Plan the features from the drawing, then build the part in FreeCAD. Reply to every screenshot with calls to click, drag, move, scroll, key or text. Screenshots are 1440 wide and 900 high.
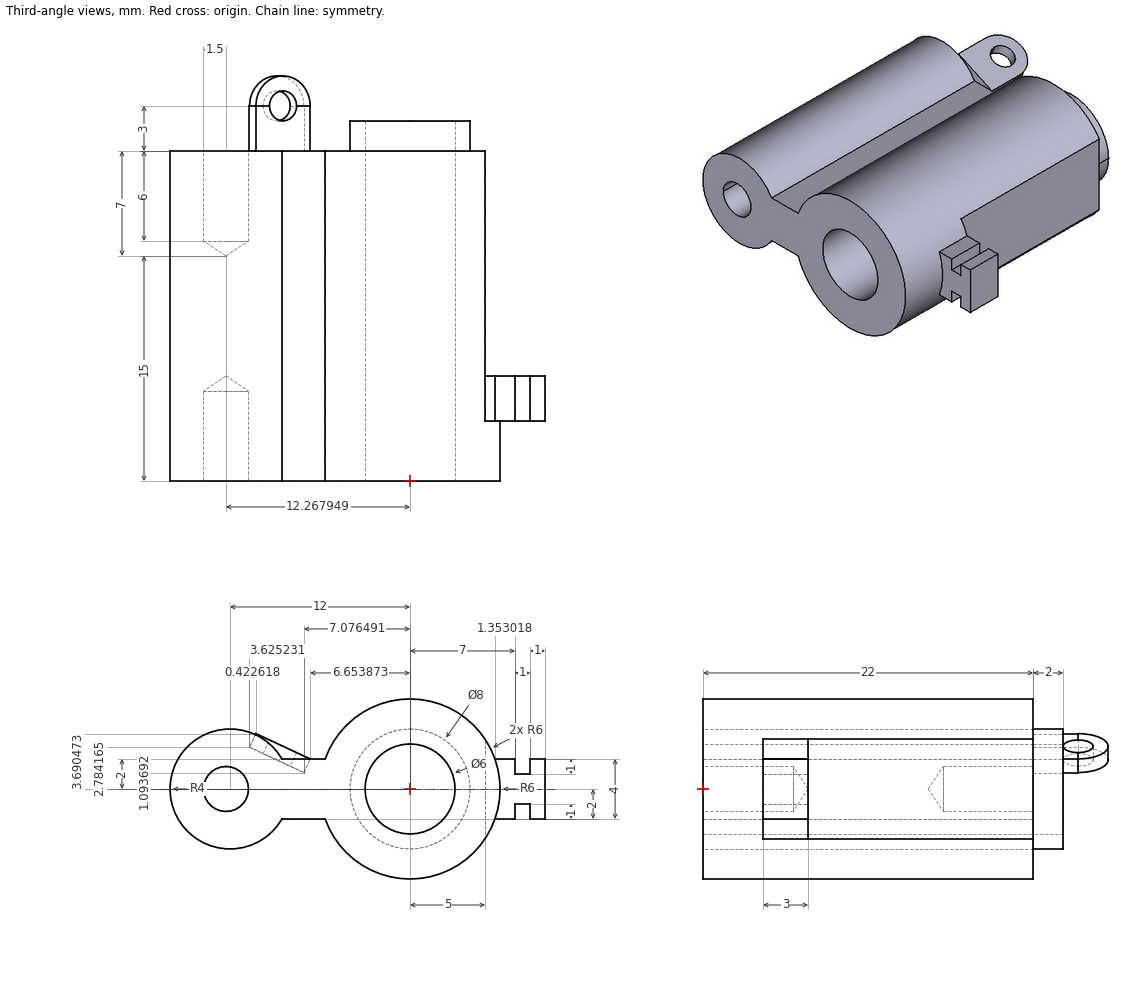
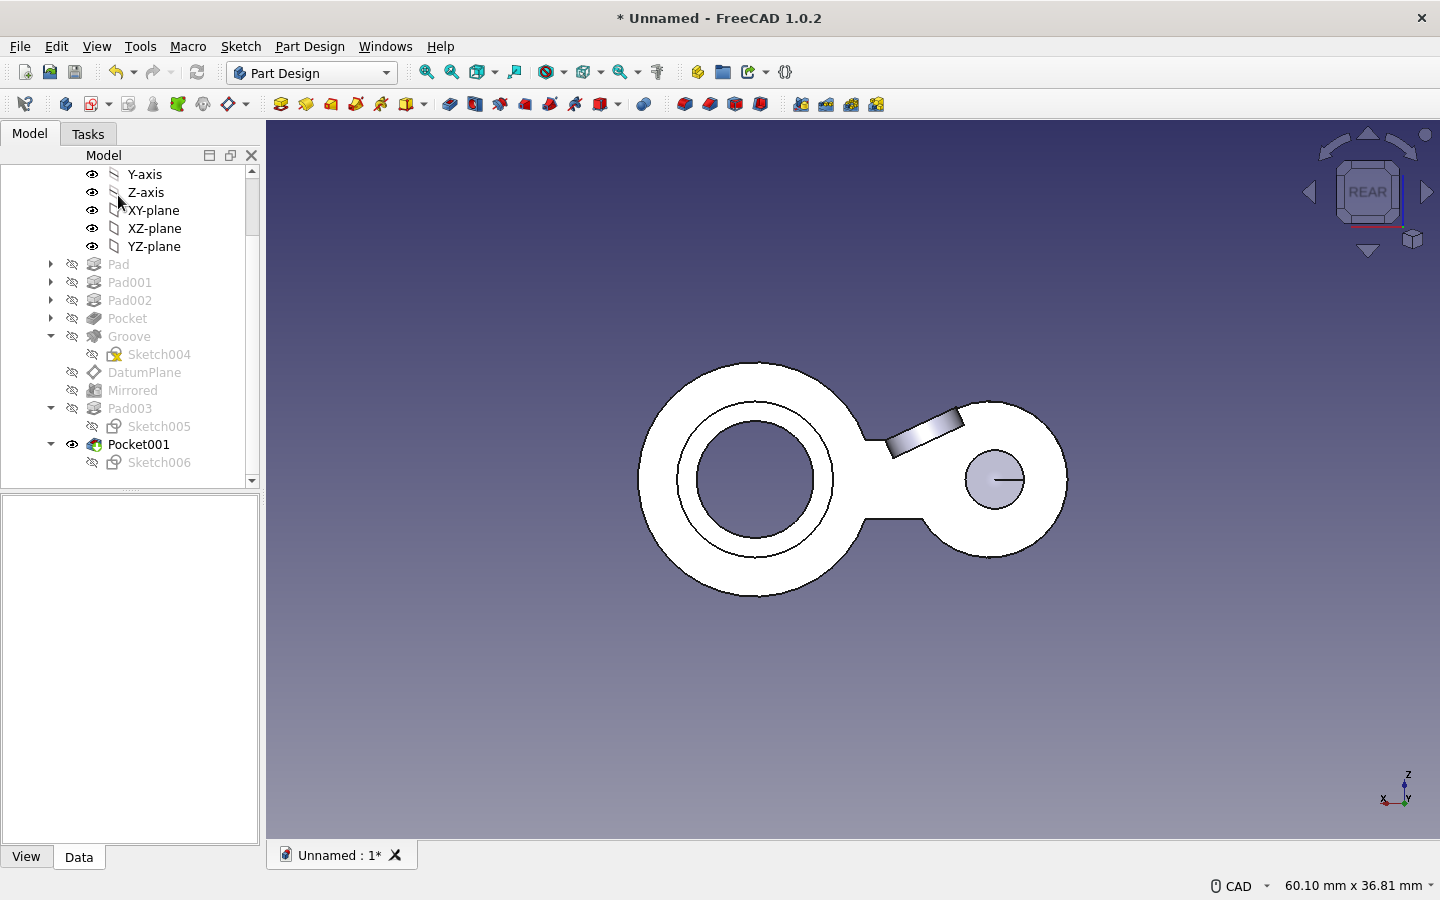
click(427, 72)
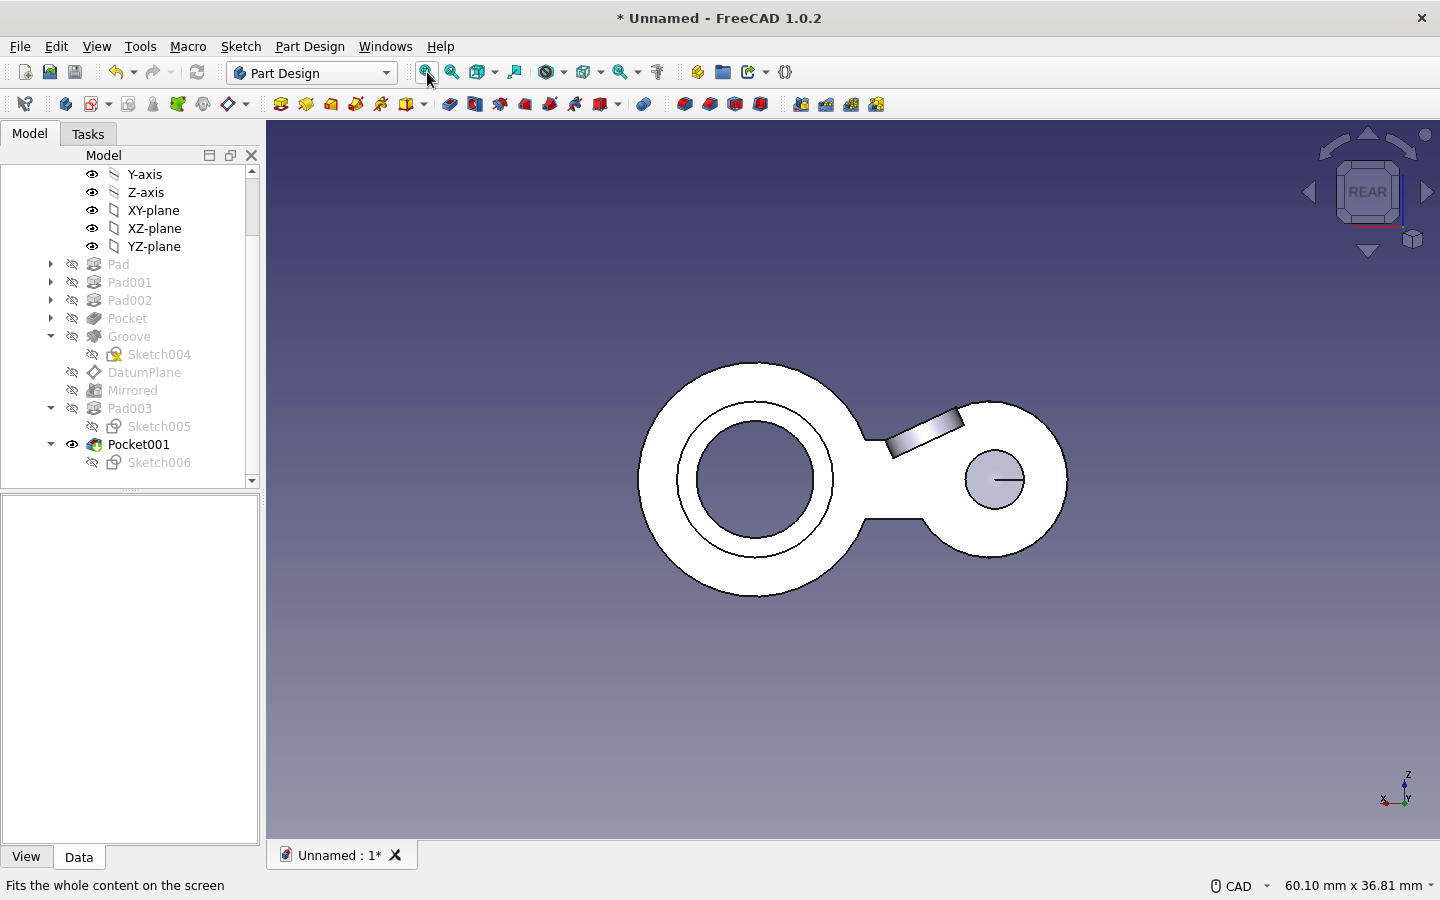
scroll(161, 314, down, 3)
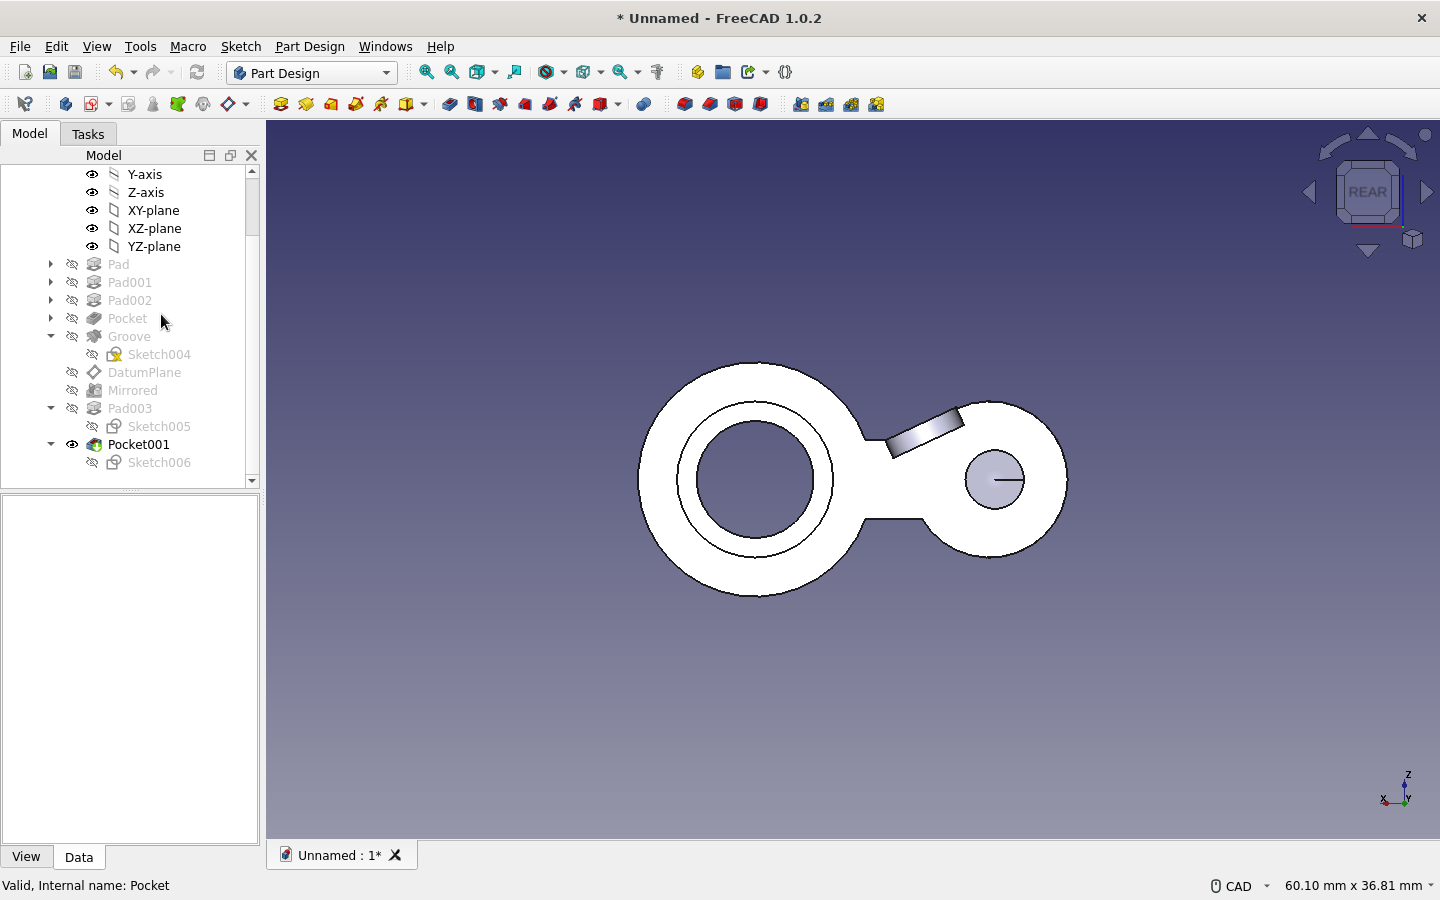
scroll(161, 314, up, 15)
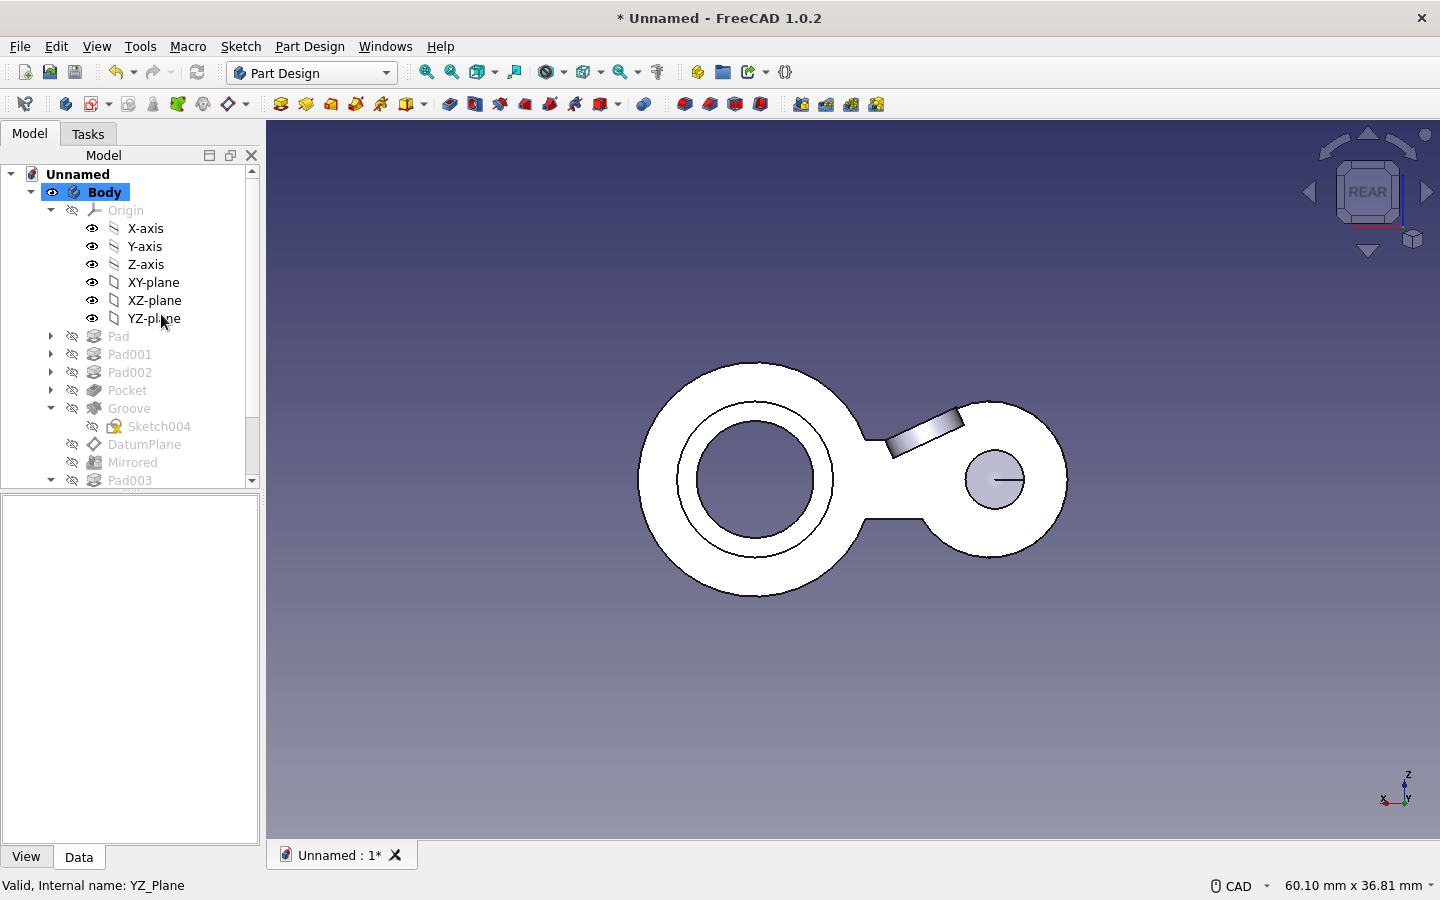
click(137, 300)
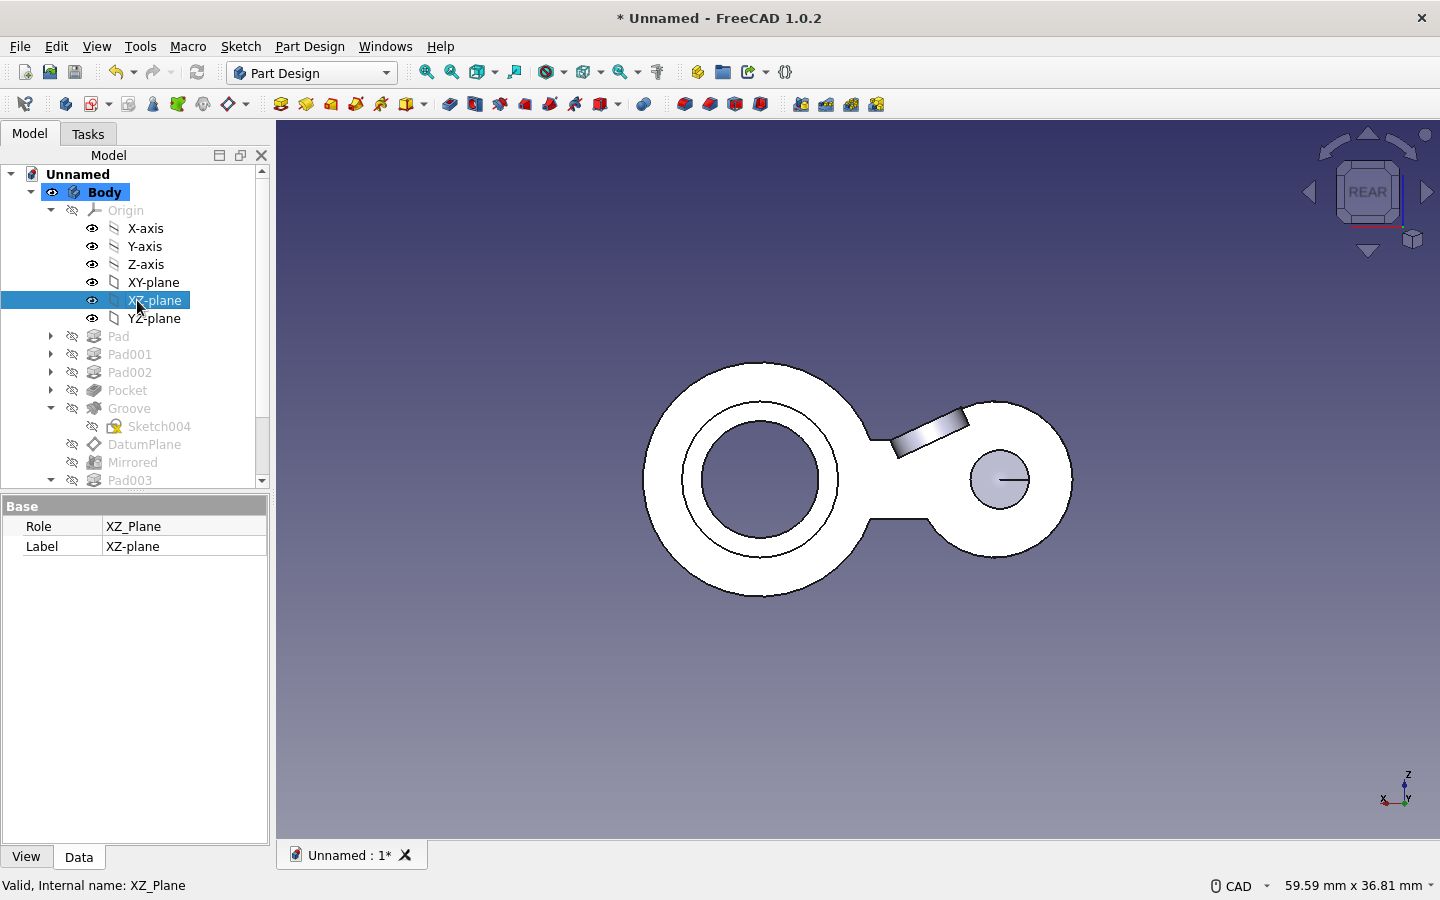
click(228, 104)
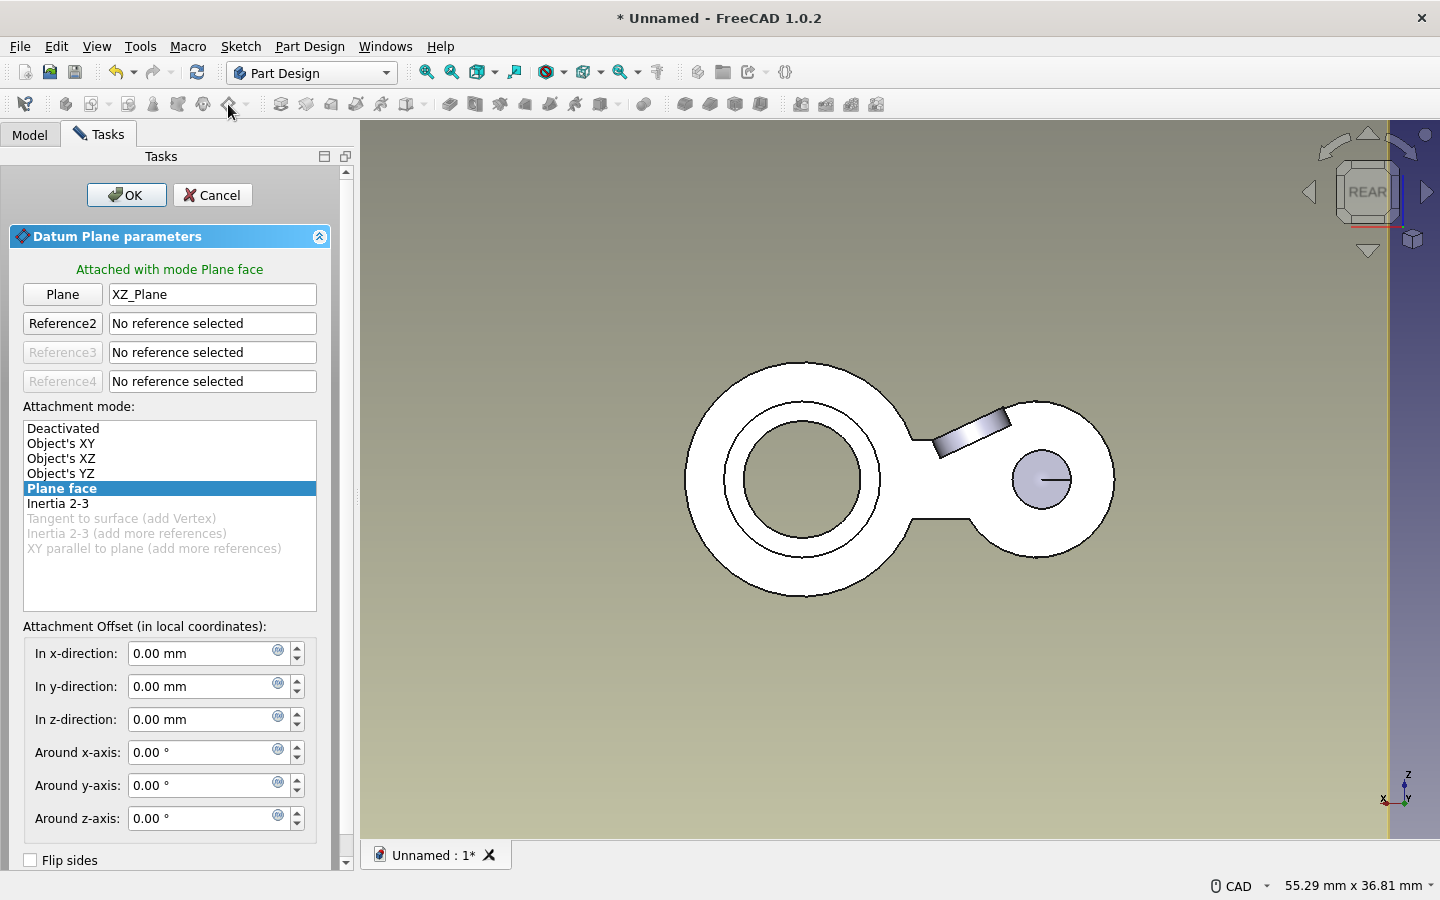
triple_click(210, 720)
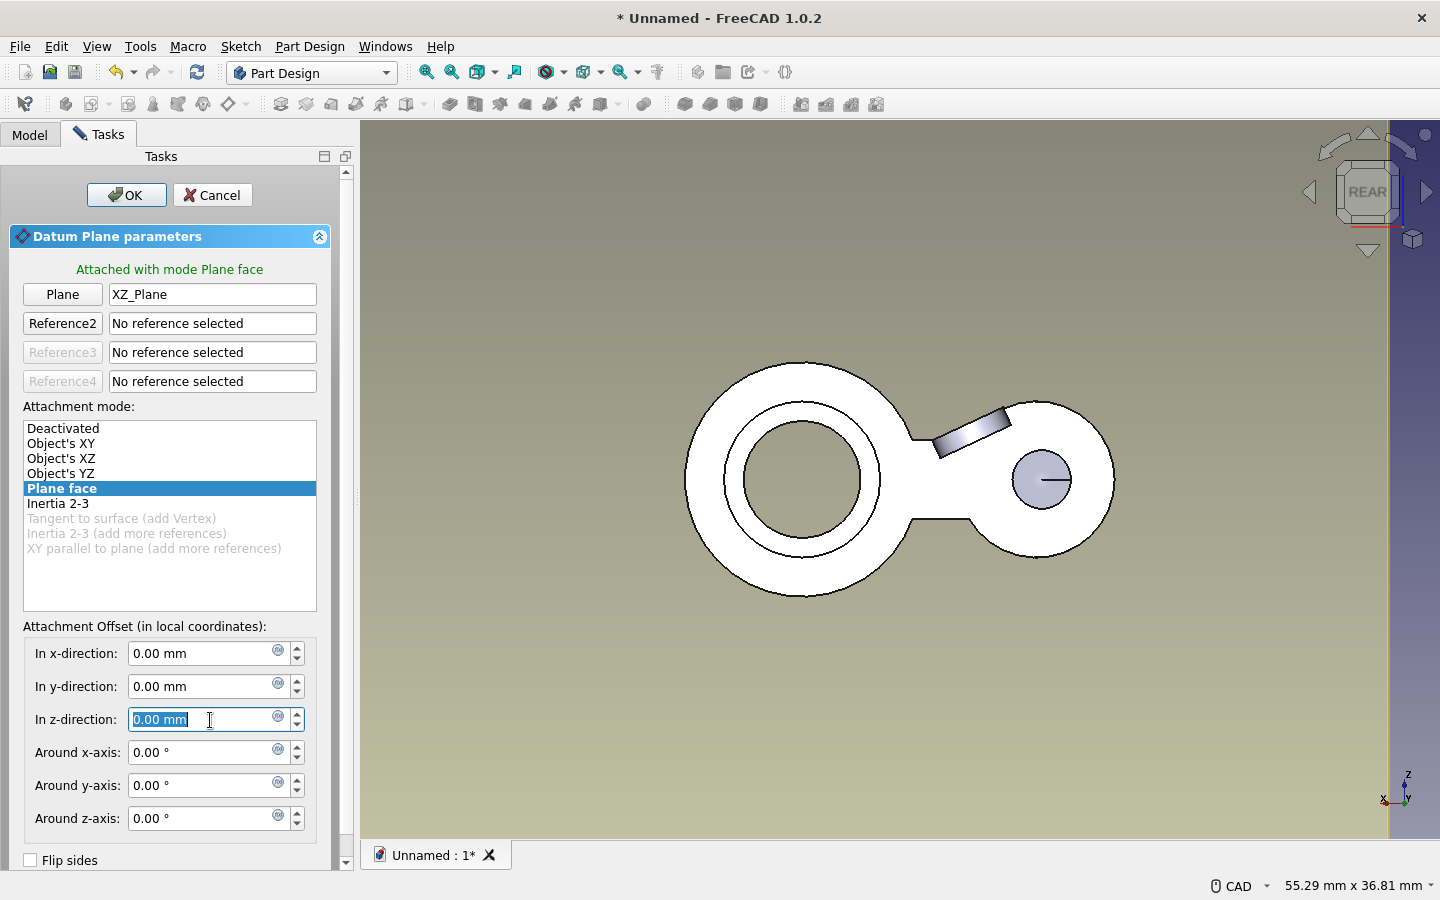
text(-4)
key(Tab)